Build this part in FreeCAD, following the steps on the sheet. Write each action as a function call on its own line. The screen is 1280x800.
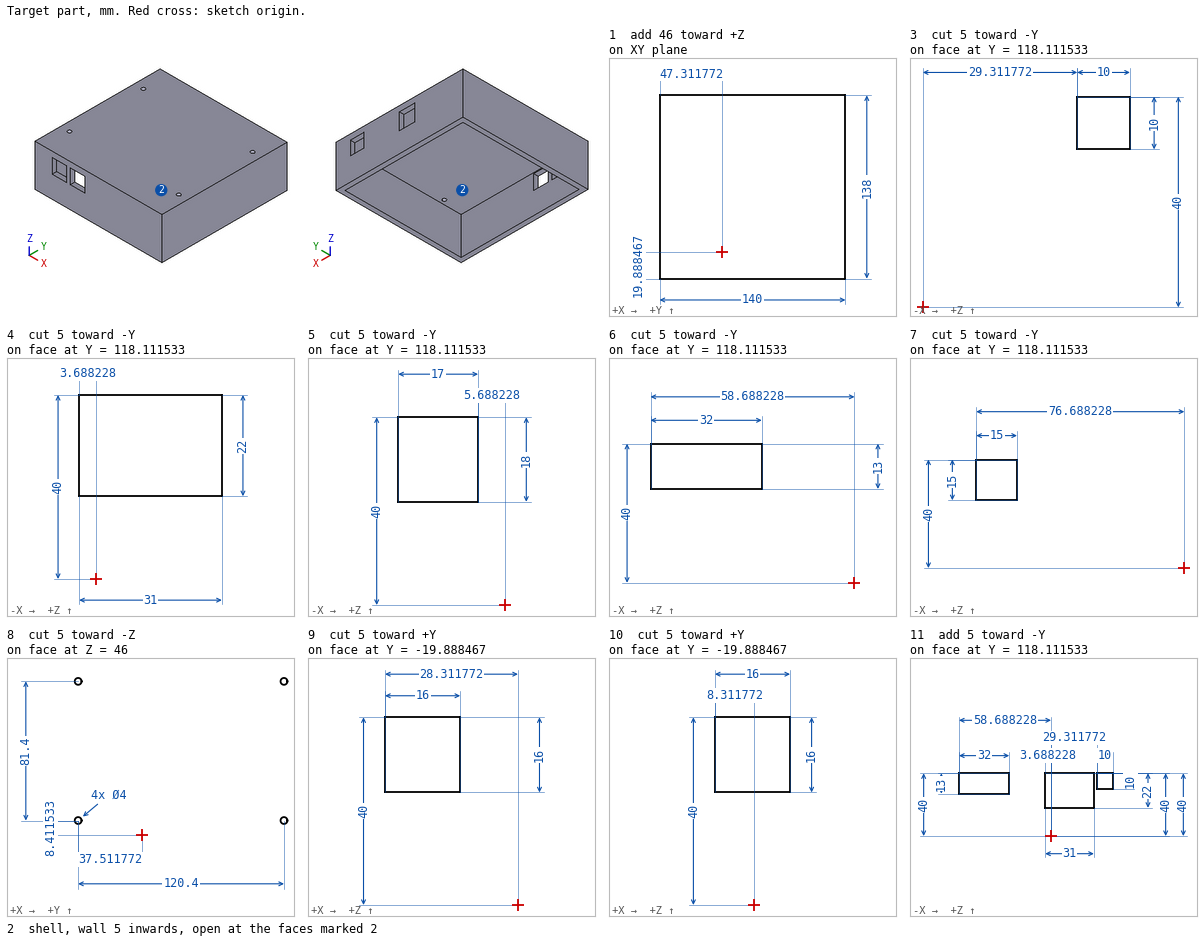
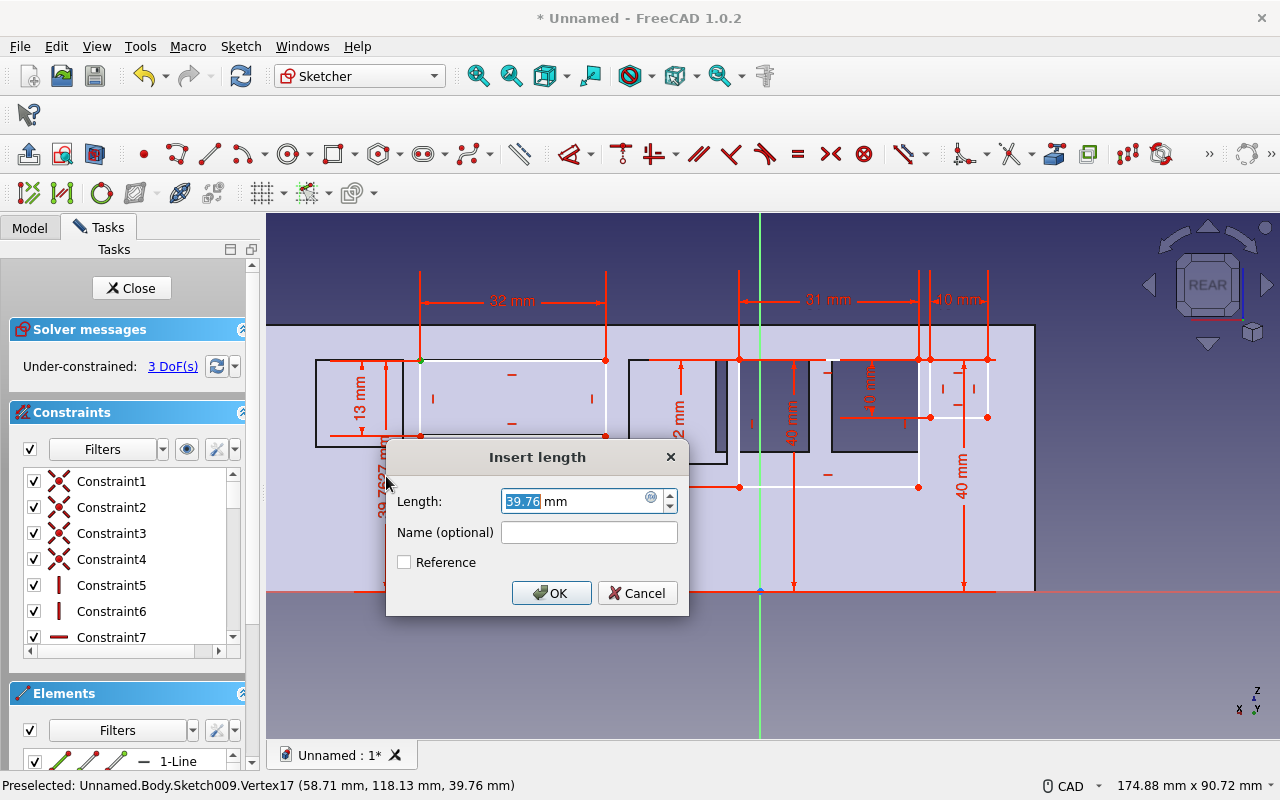
text(40)
key(Return)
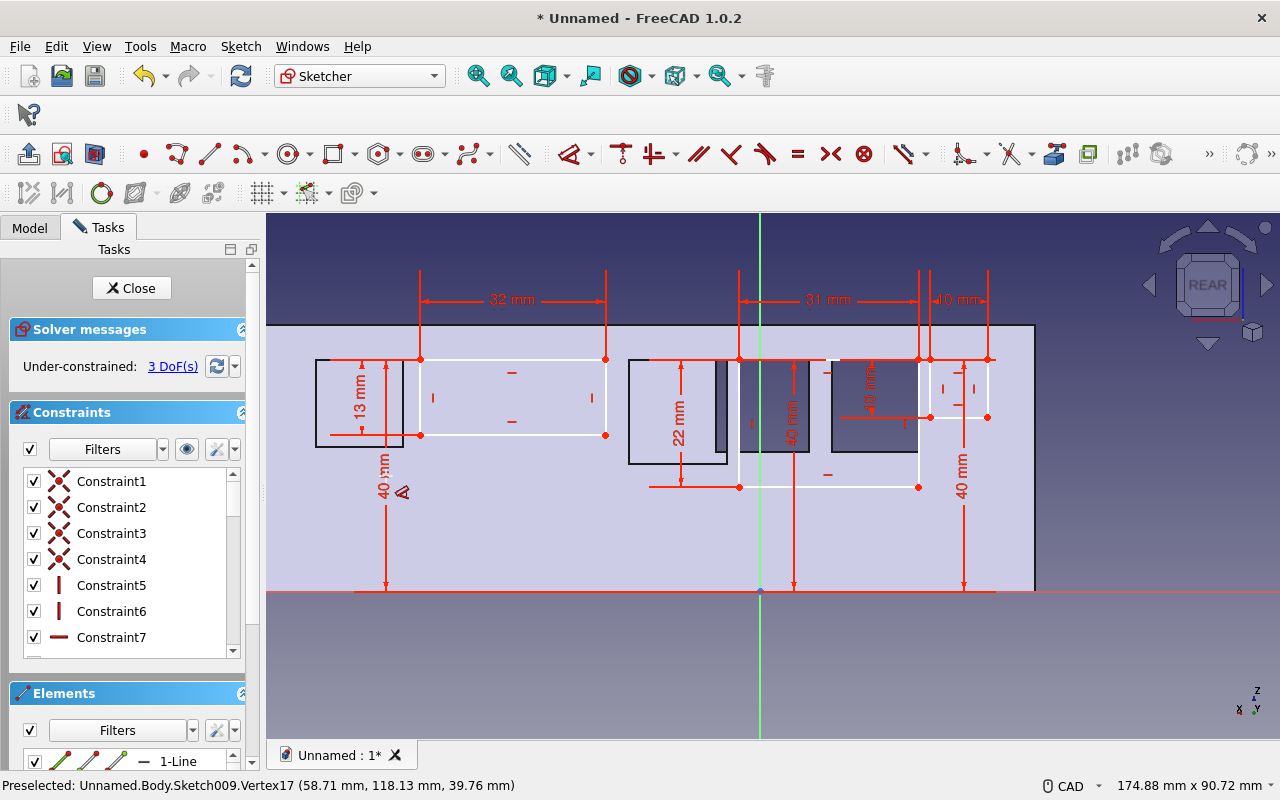
scroll(739, 360, up, 4)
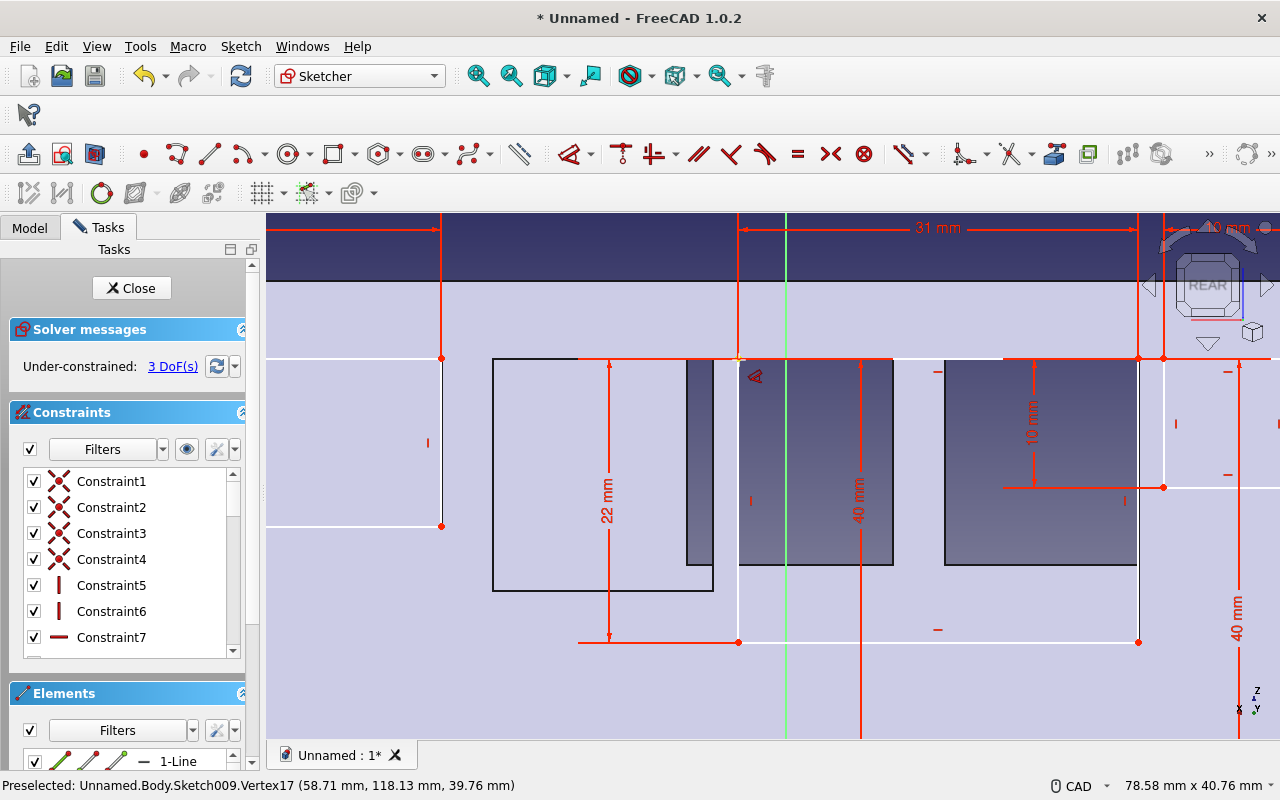
click(738, 359)
click(762, 325)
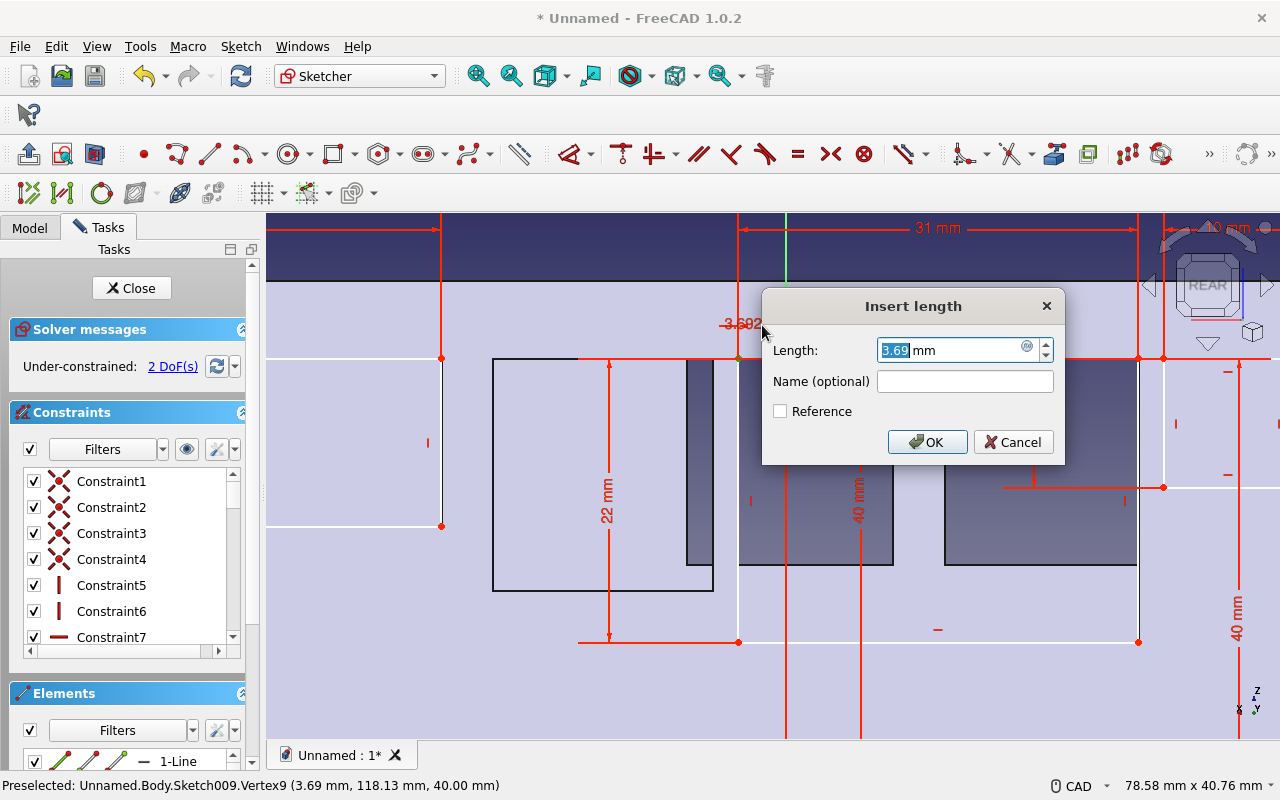
text(3.688228)
key(Return)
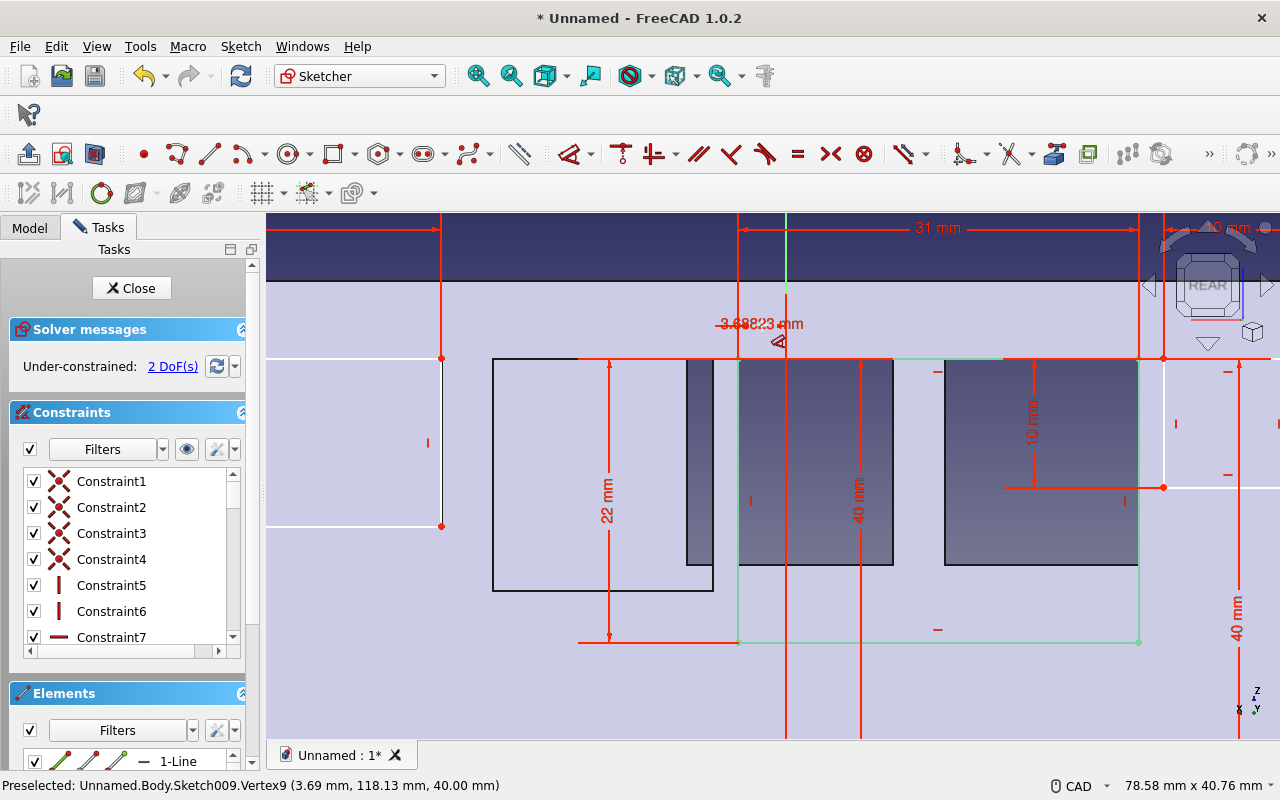
scroll(740, 361, down, 4)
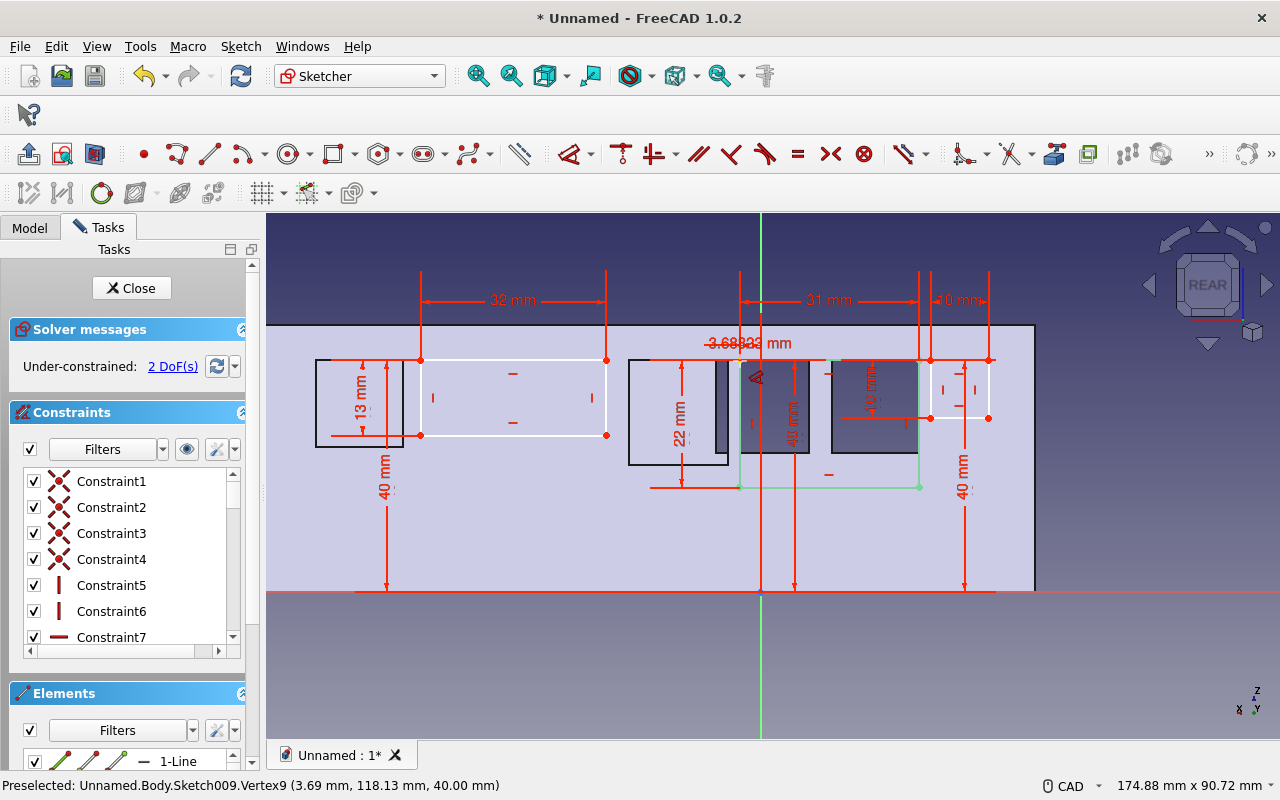
click(931, 360)
click(846, 626)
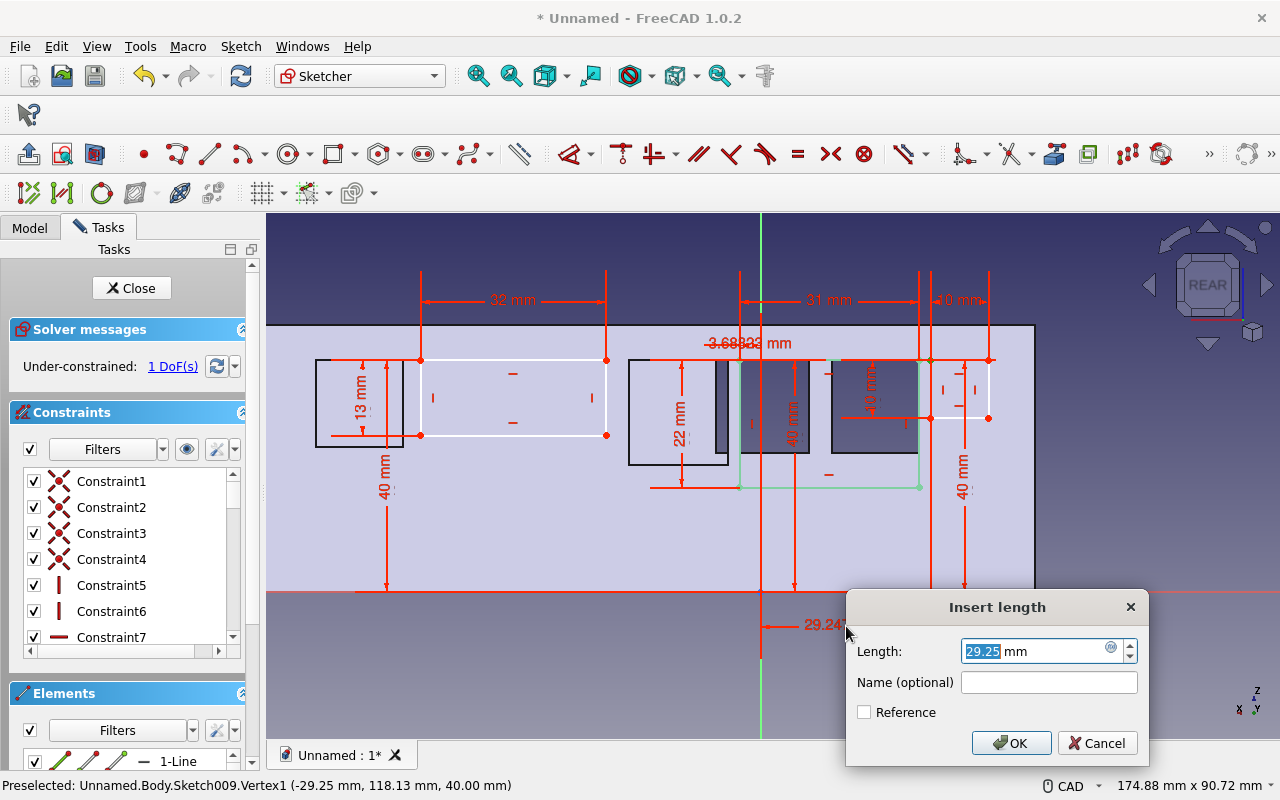
text(29.311772)
key(Return)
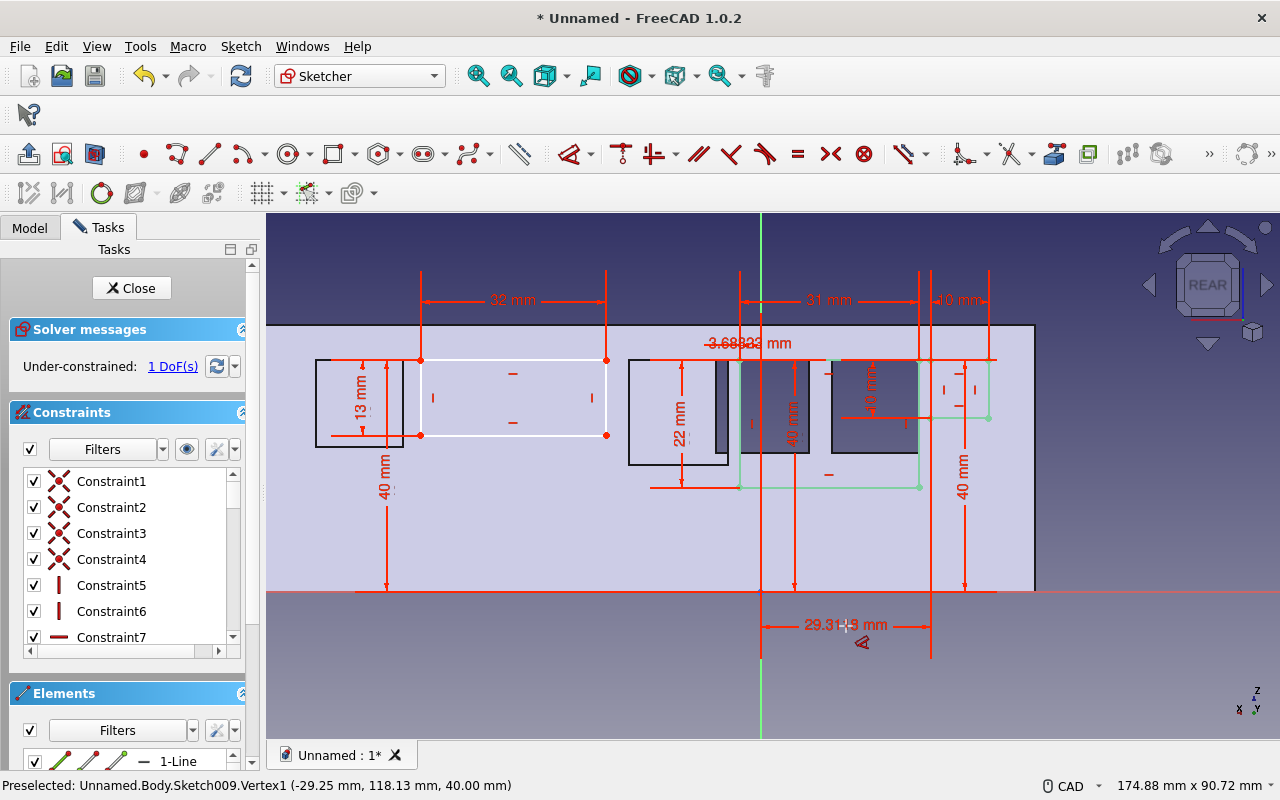
click(421, 360)
click(591, 626)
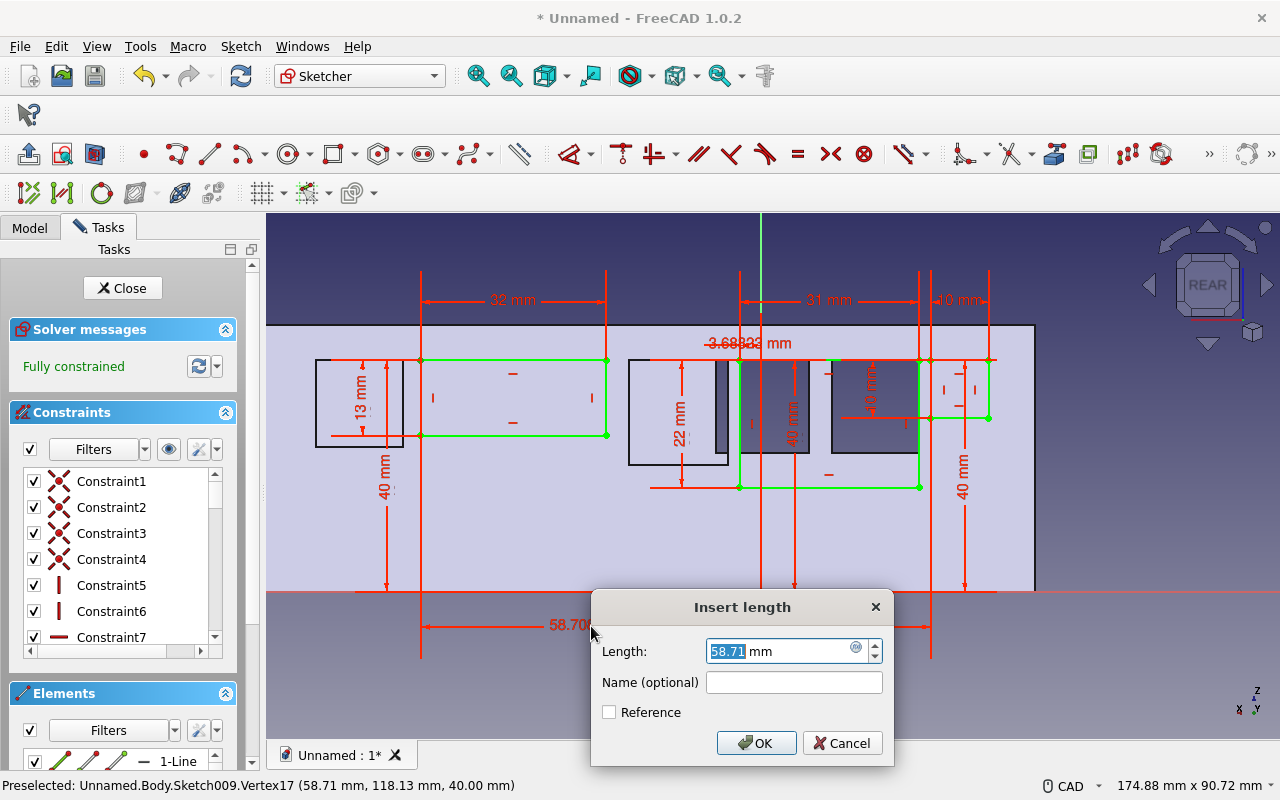
text(58.688228)
key(Return)
key(Escape)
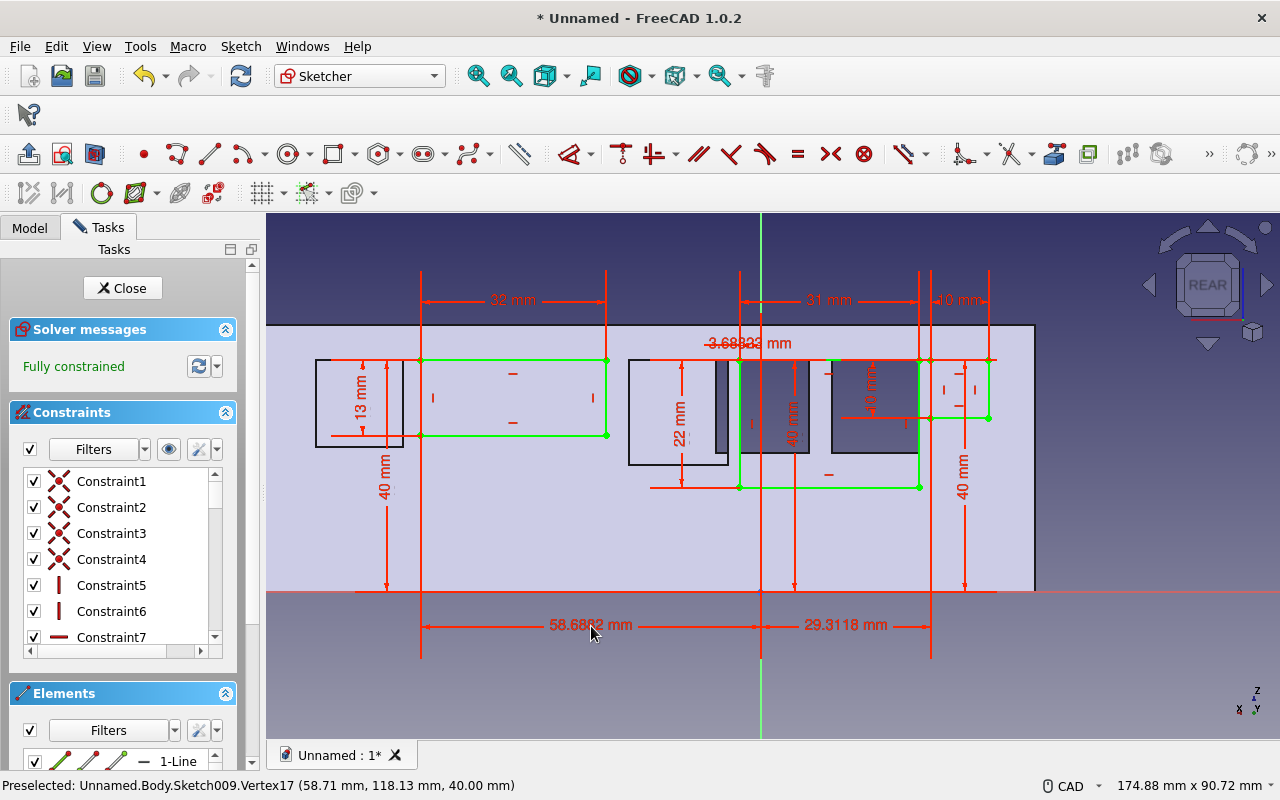
click(123, 288)